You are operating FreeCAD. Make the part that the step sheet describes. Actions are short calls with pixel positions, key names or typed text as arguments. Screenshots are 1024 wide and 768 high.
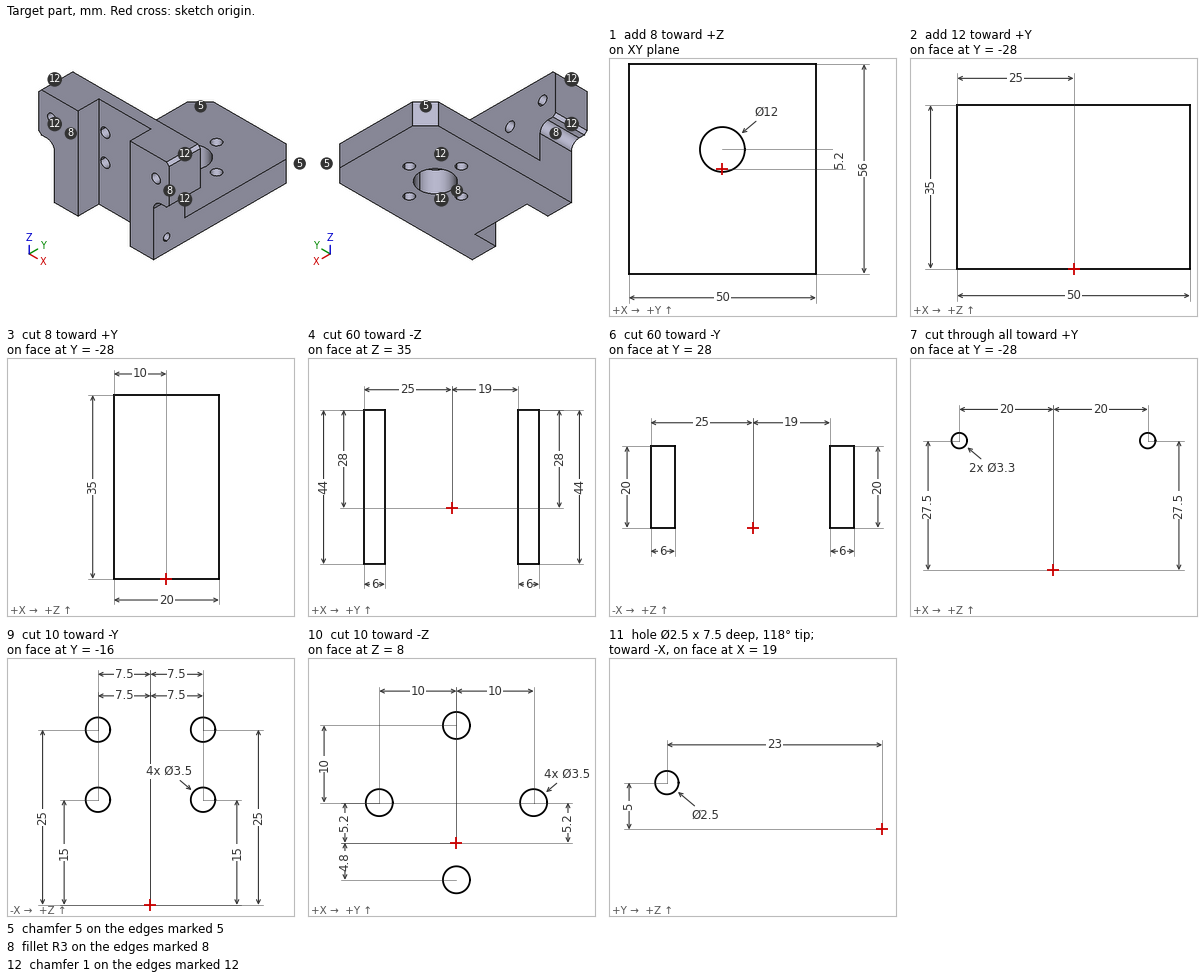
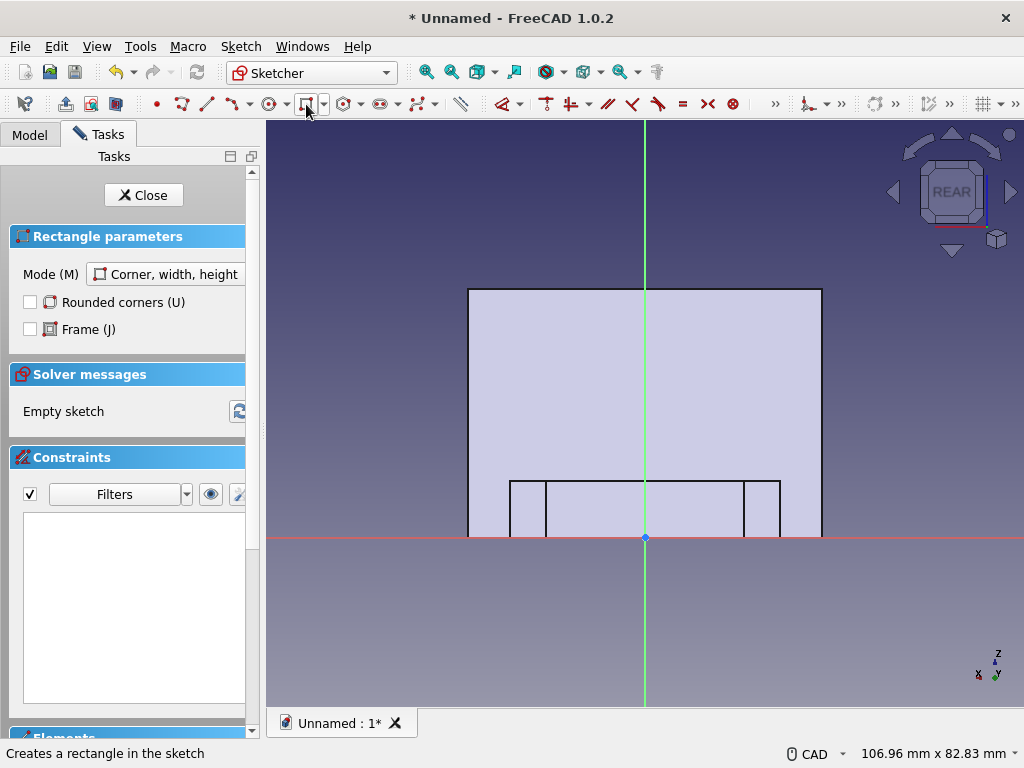
click(780, 396)
click(822, 538)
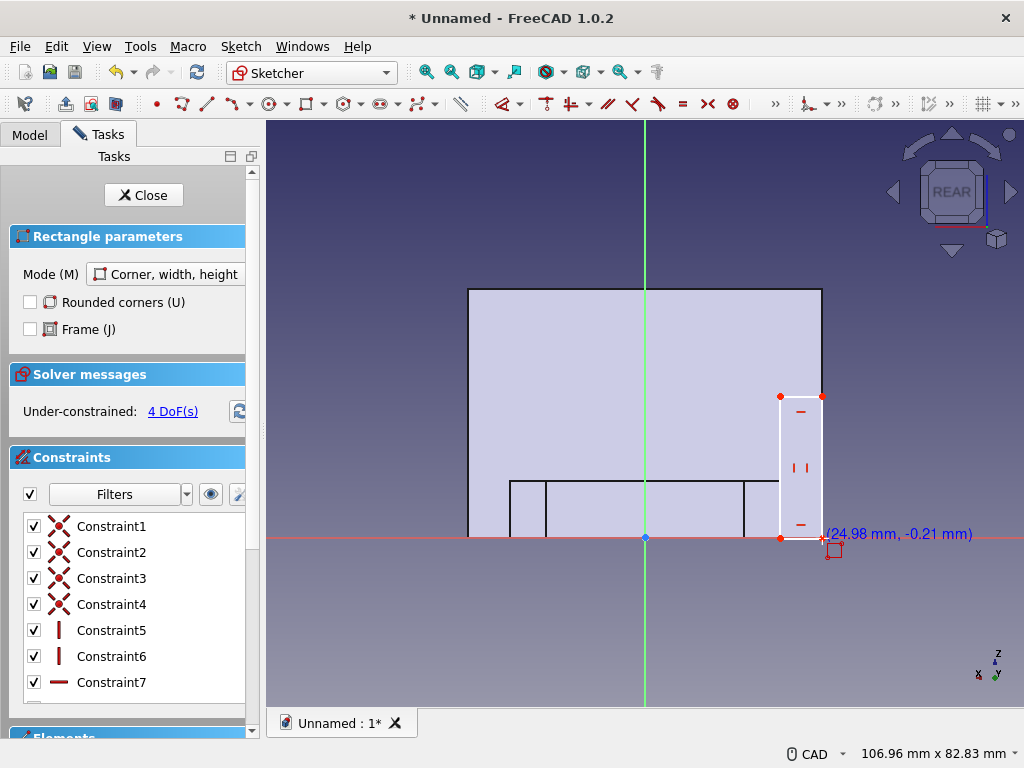
click(468, 396)
click(510, 538)
key(Escape)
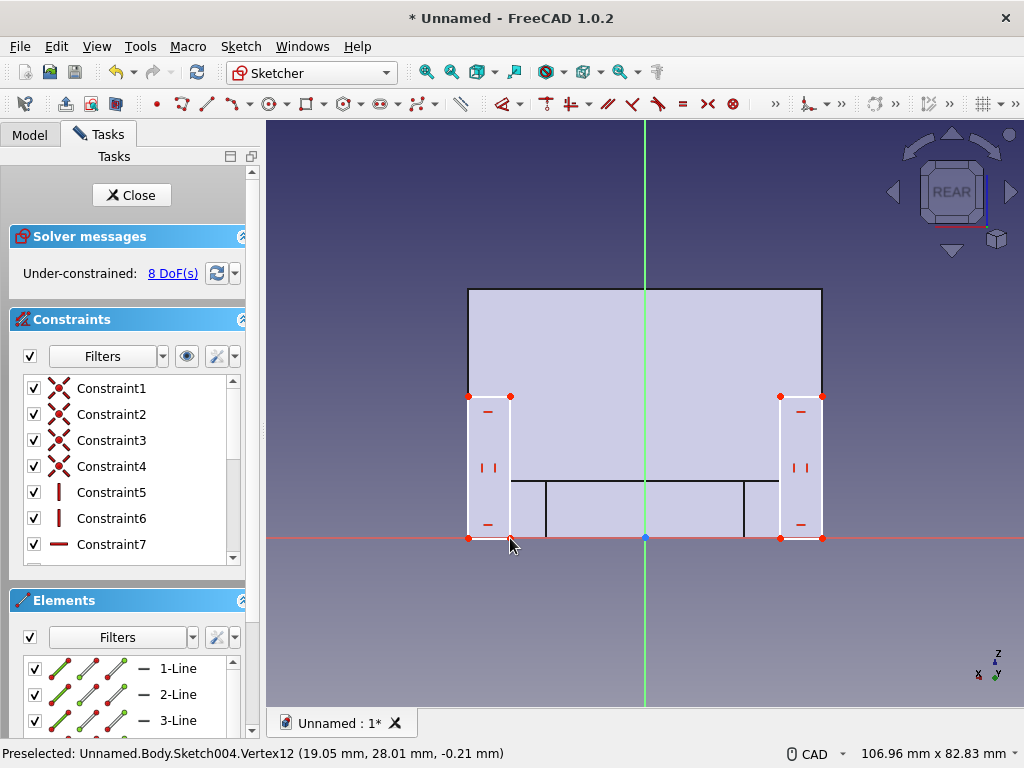
click(780, 539)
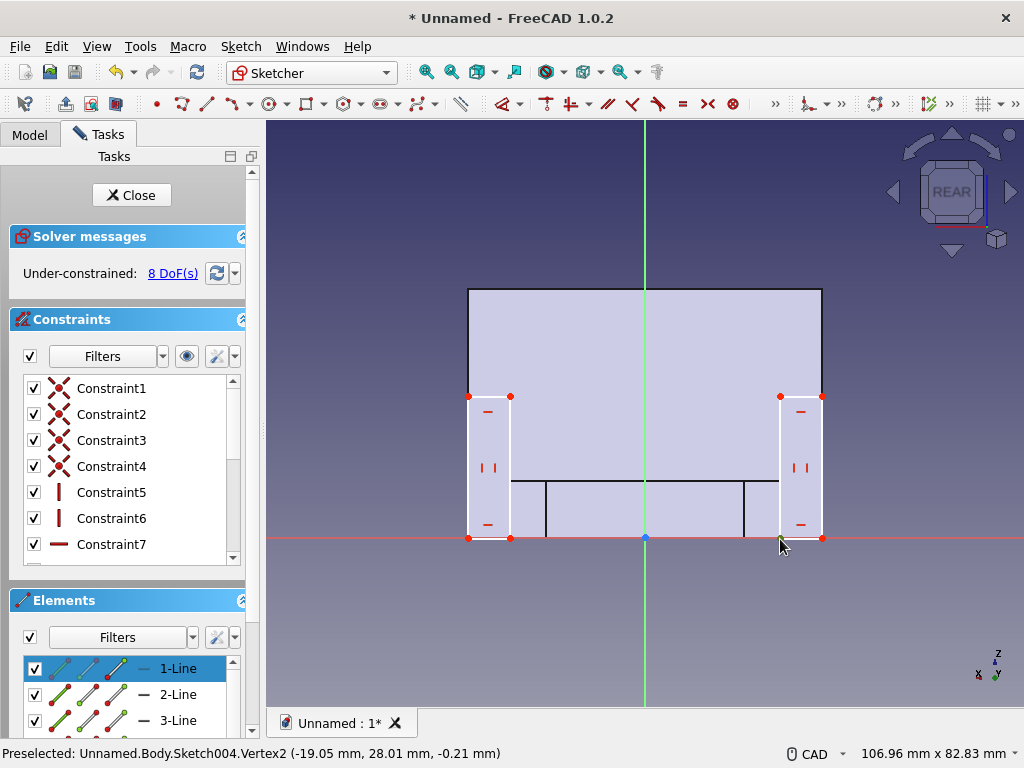
click(334, 538)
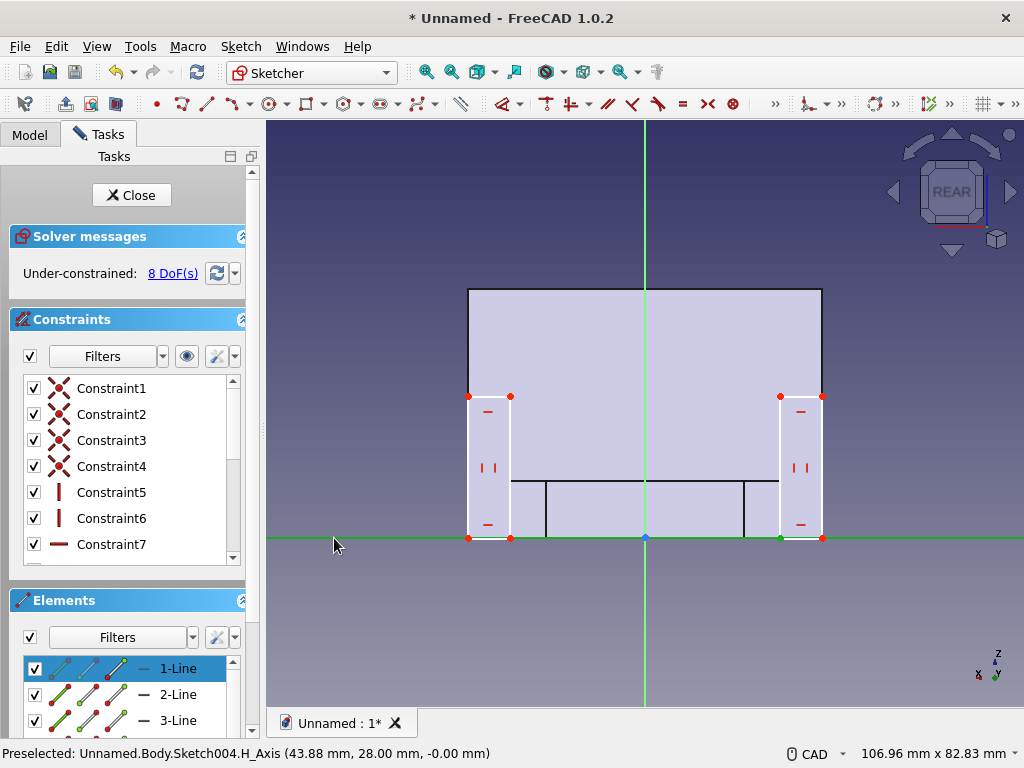
click(546, 104)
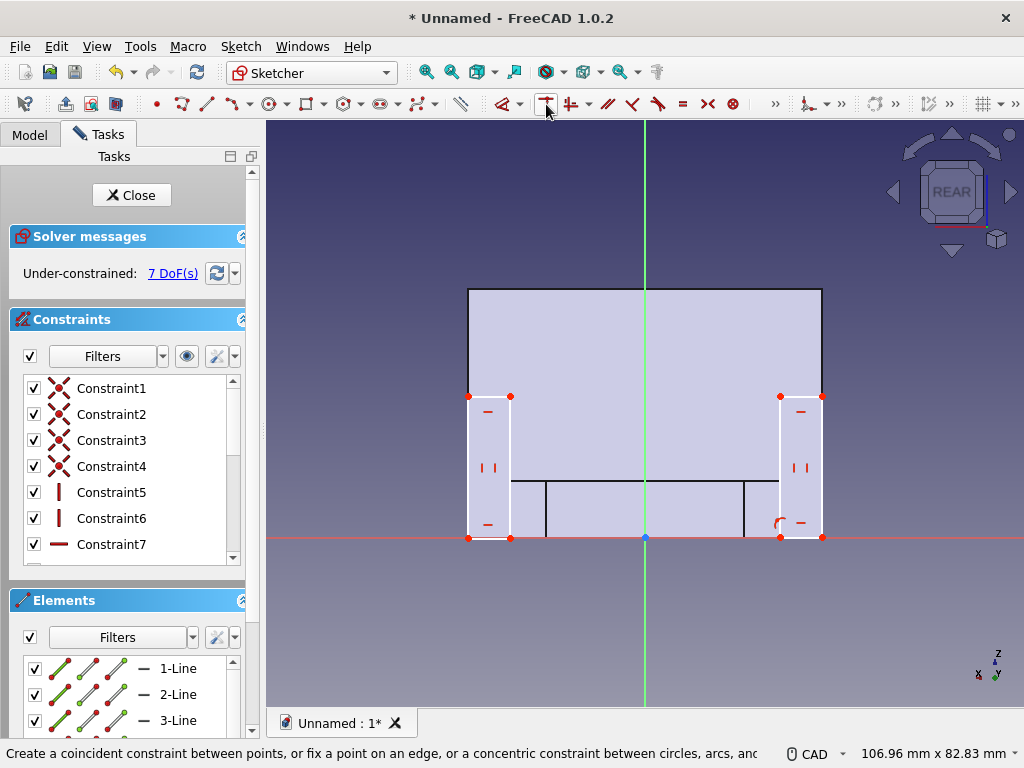
click(468, 539)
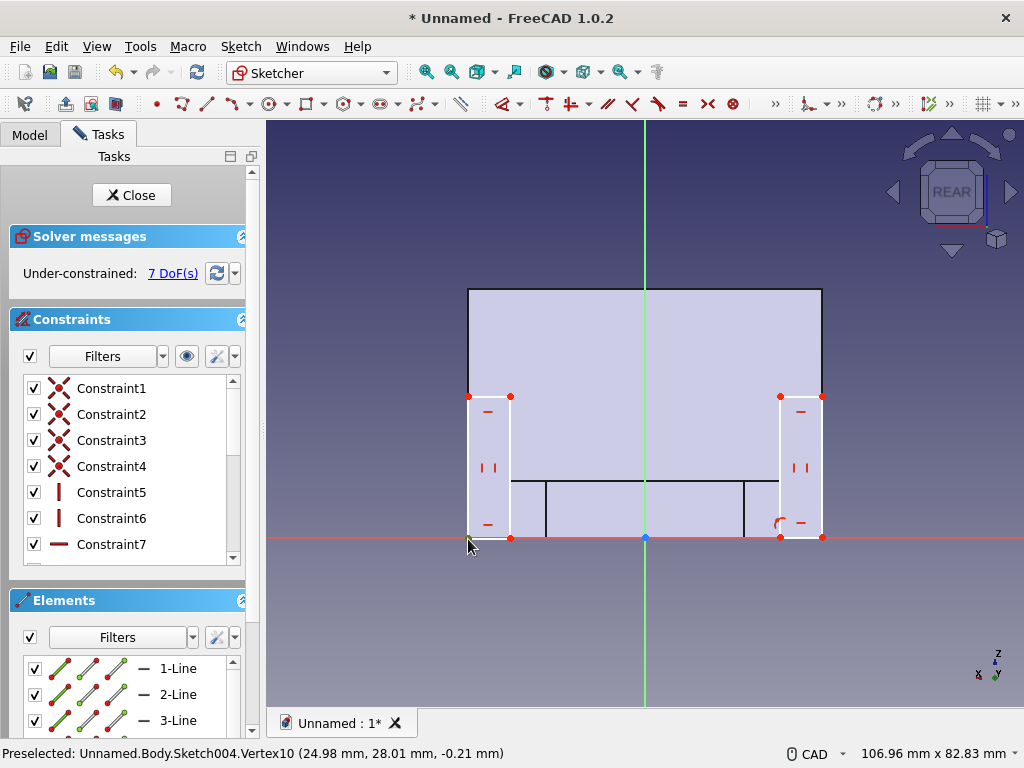
click(334, 538)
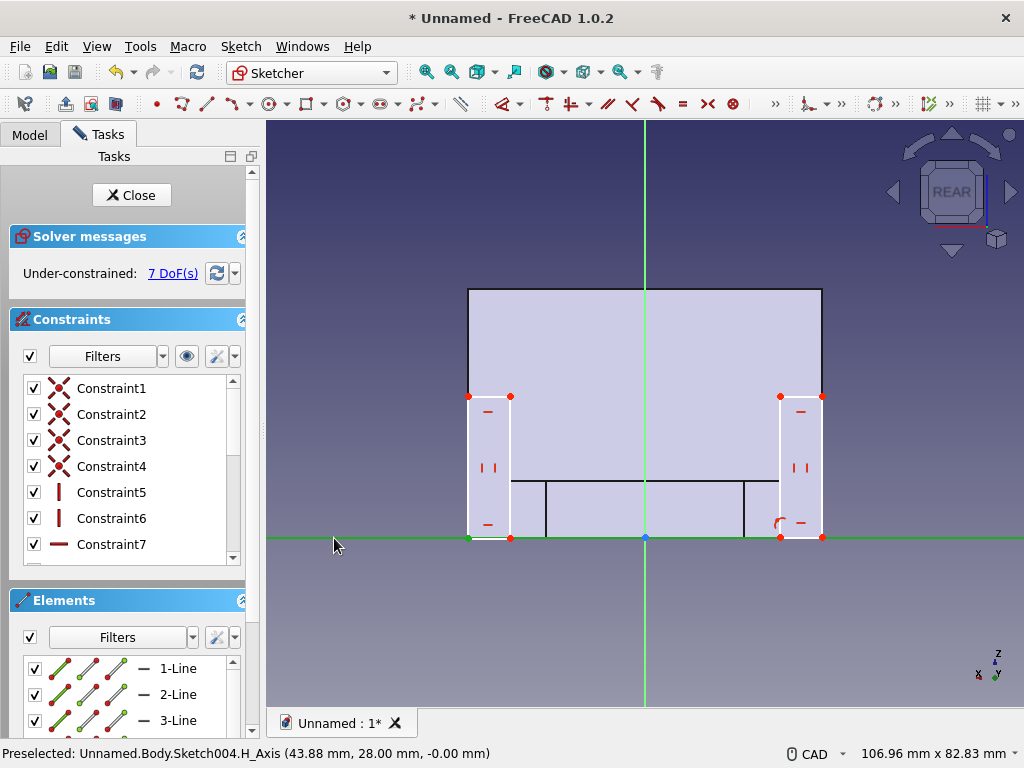
click(546, 104)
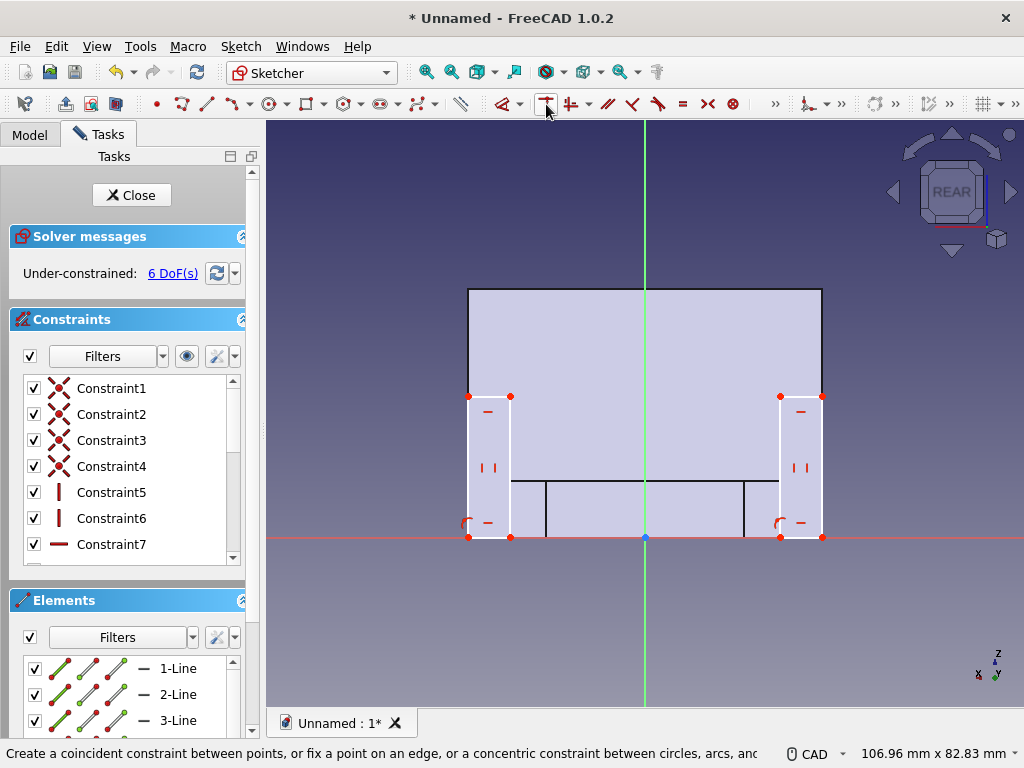
click(502, 104)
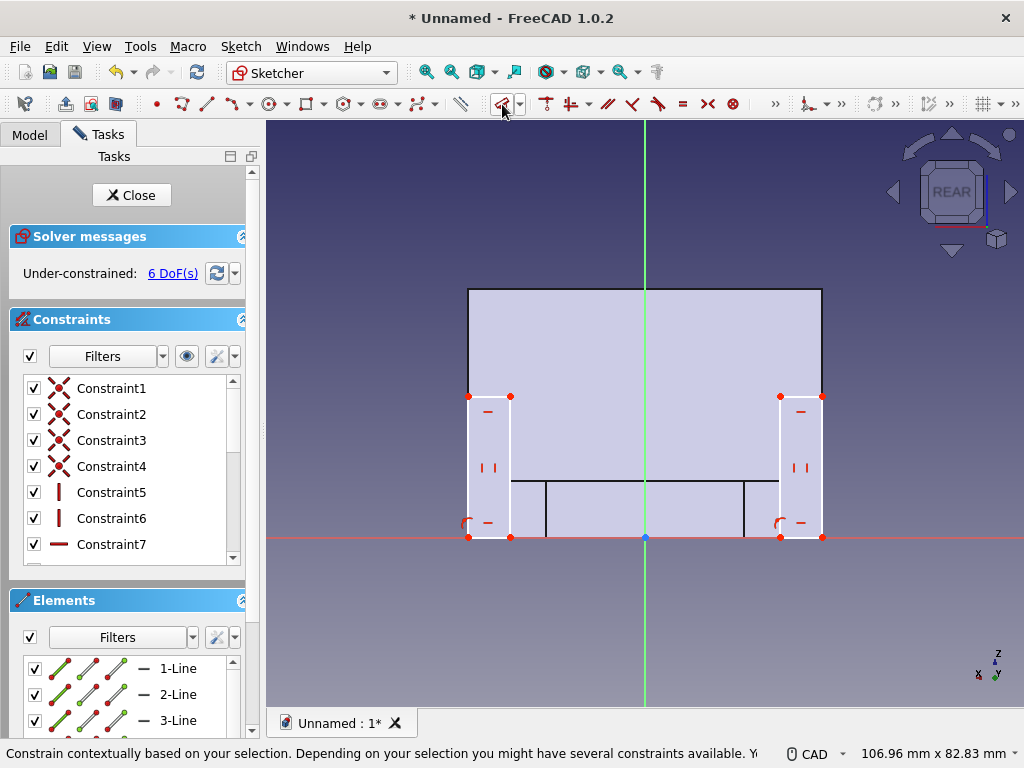
click(793, 538)
click(801, 572)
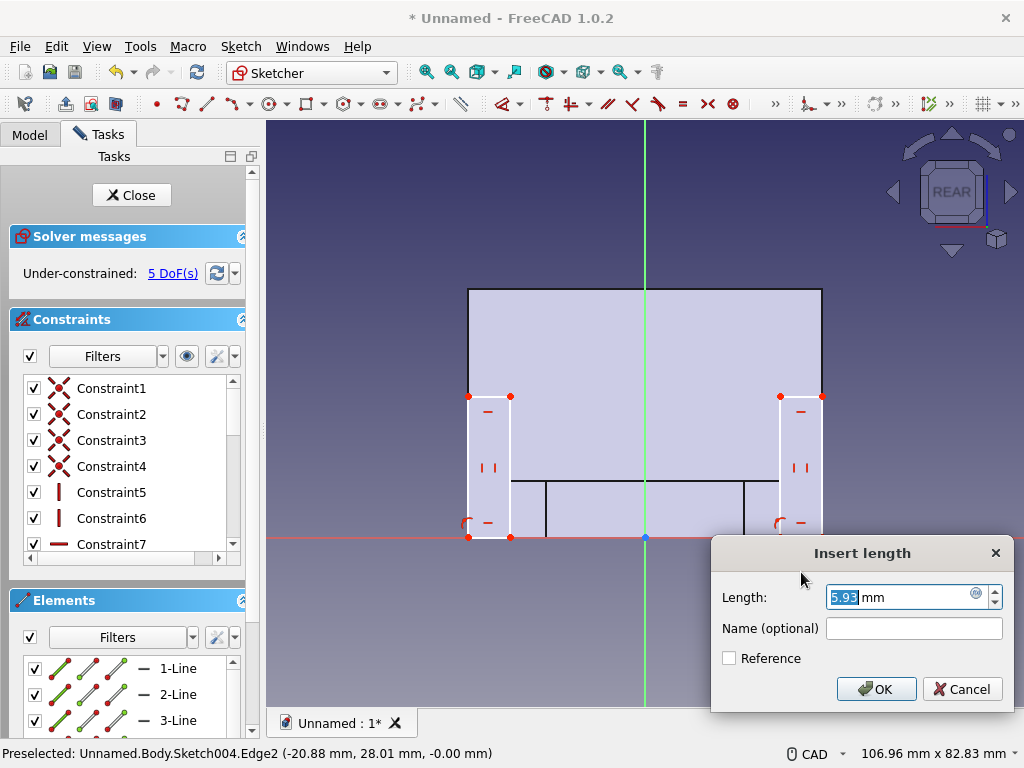
text(6)
key(Return)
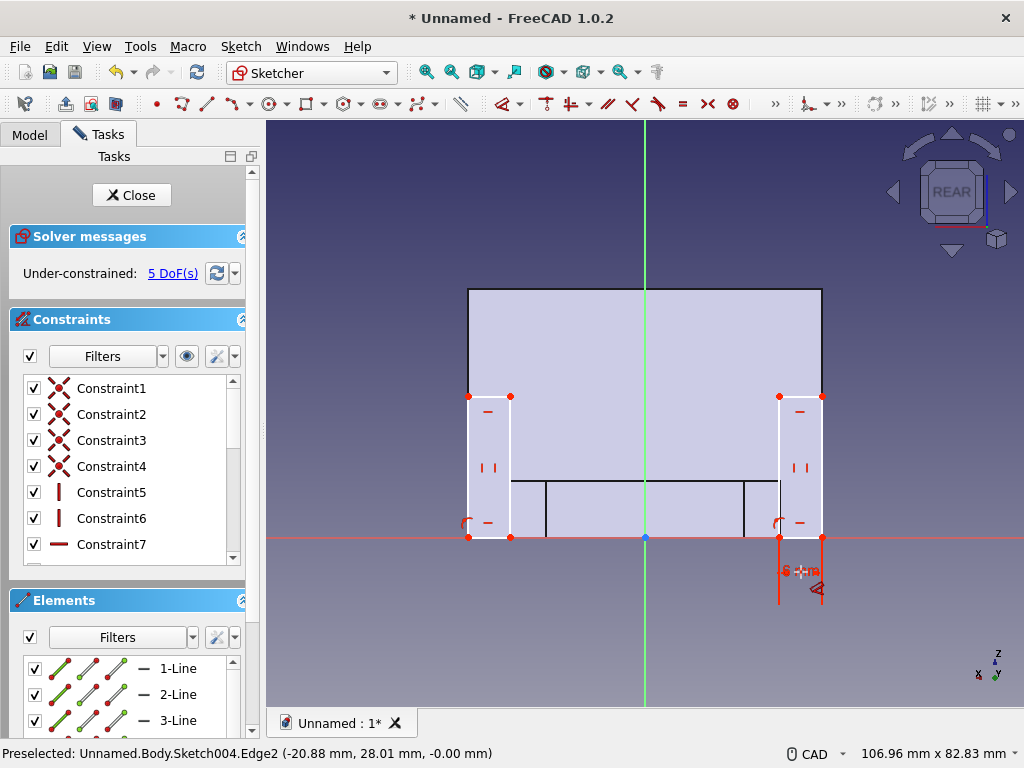
click(481, 538)
click(489, 572)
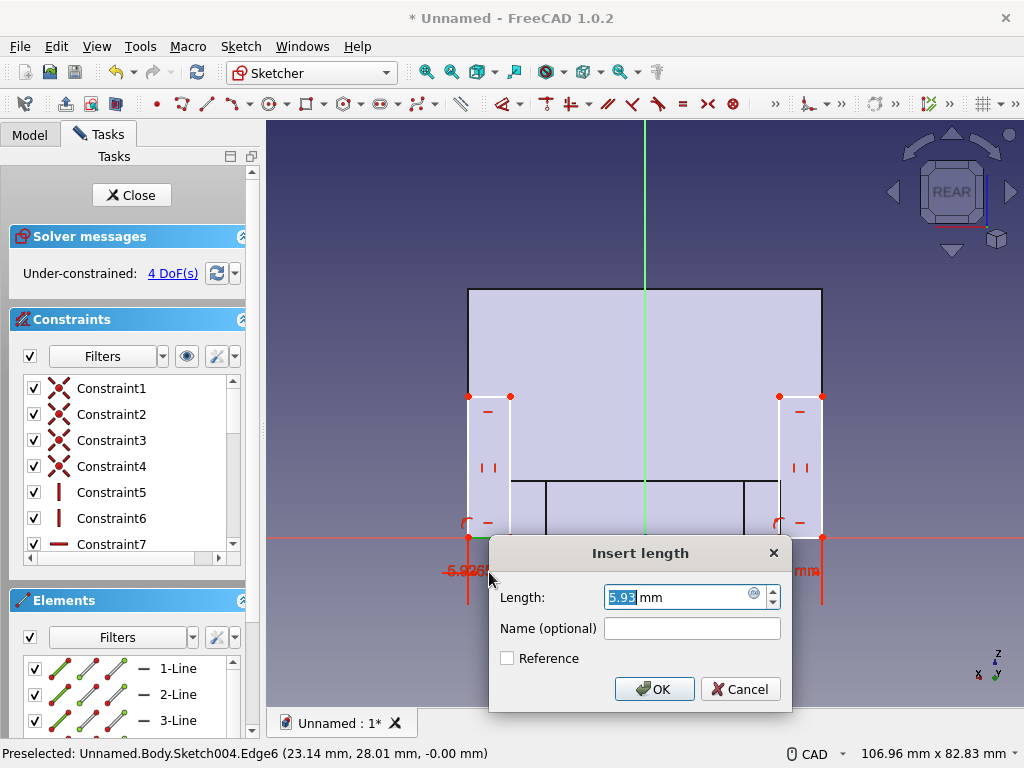
text(6)
key(Return)